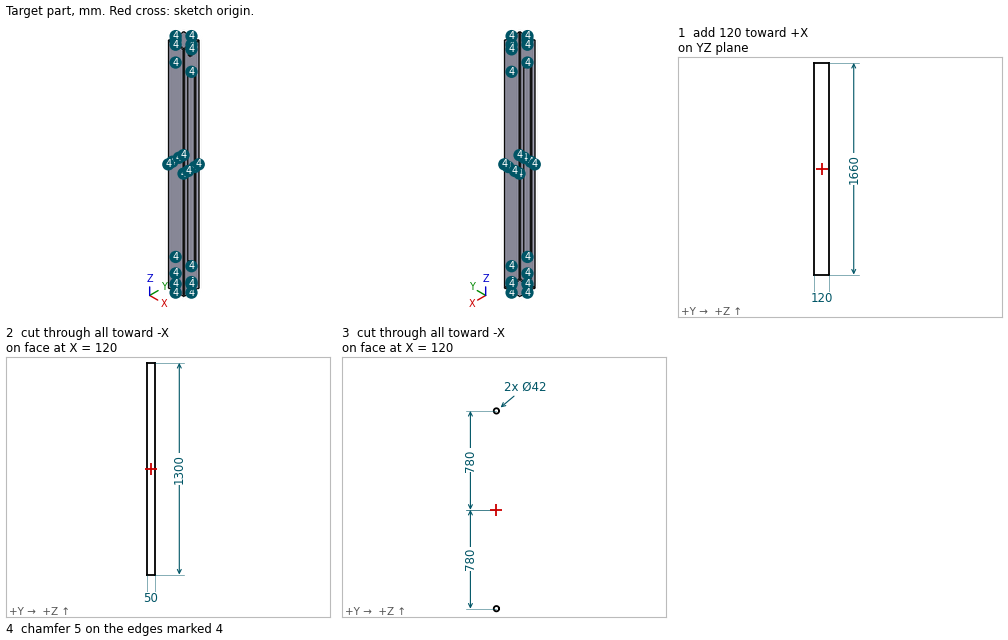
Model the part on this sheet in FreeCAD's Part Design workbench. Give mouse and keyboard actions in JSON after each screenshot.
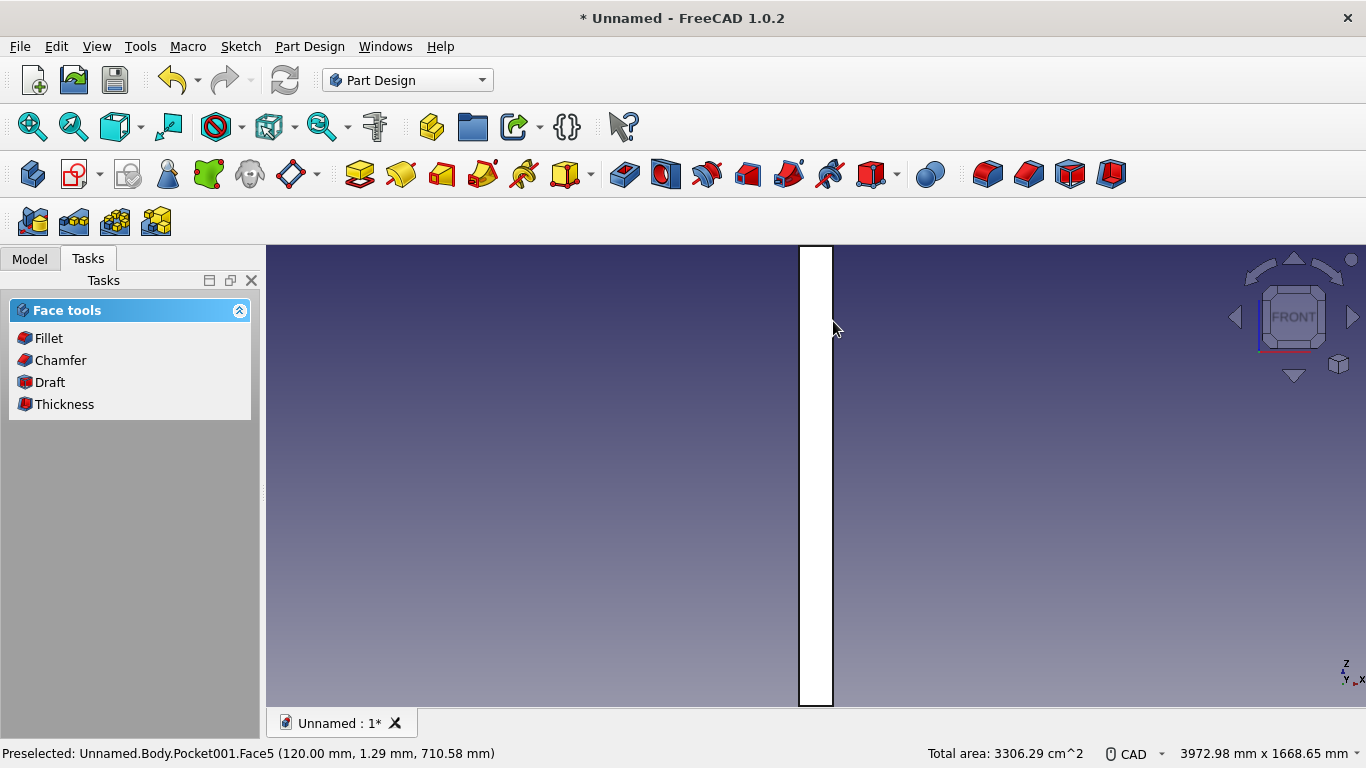
{"action": "key", "text": "3"}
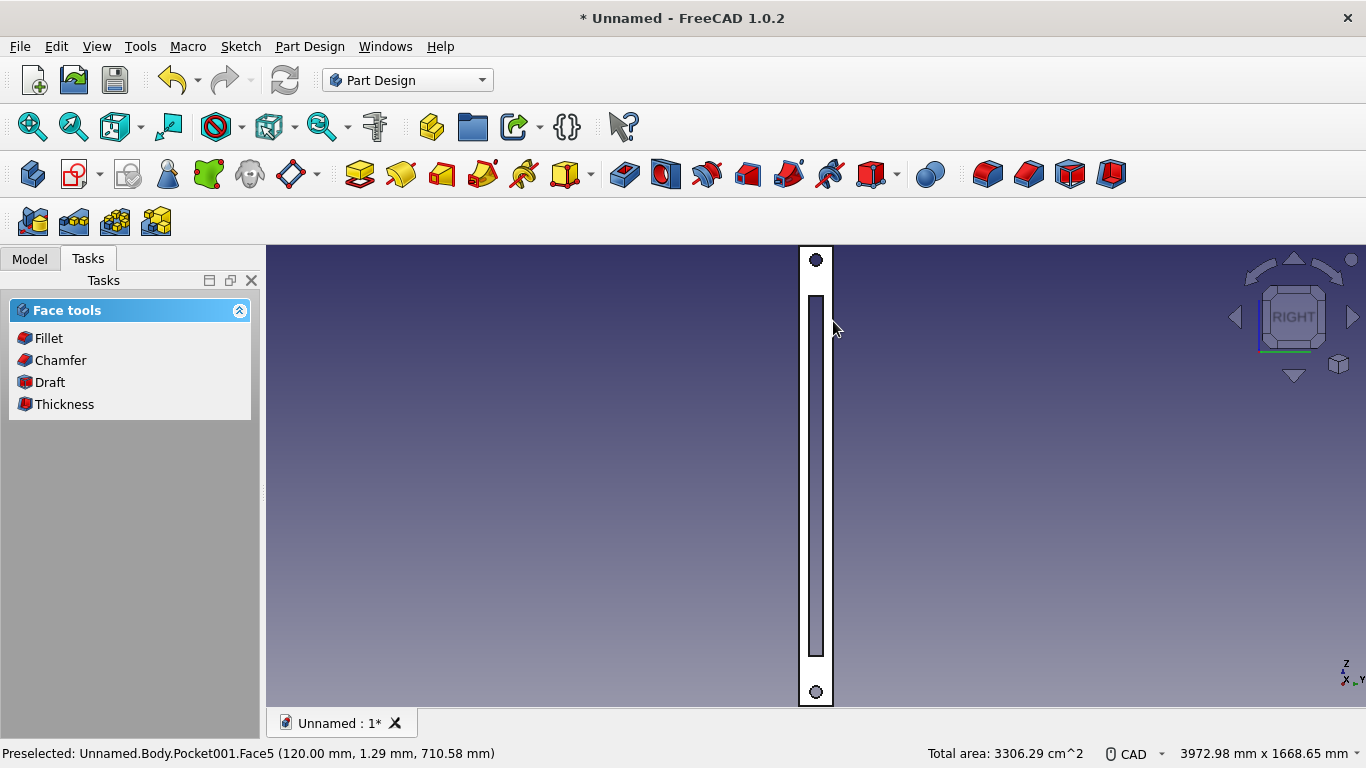
{"action": "key", "text": "5"}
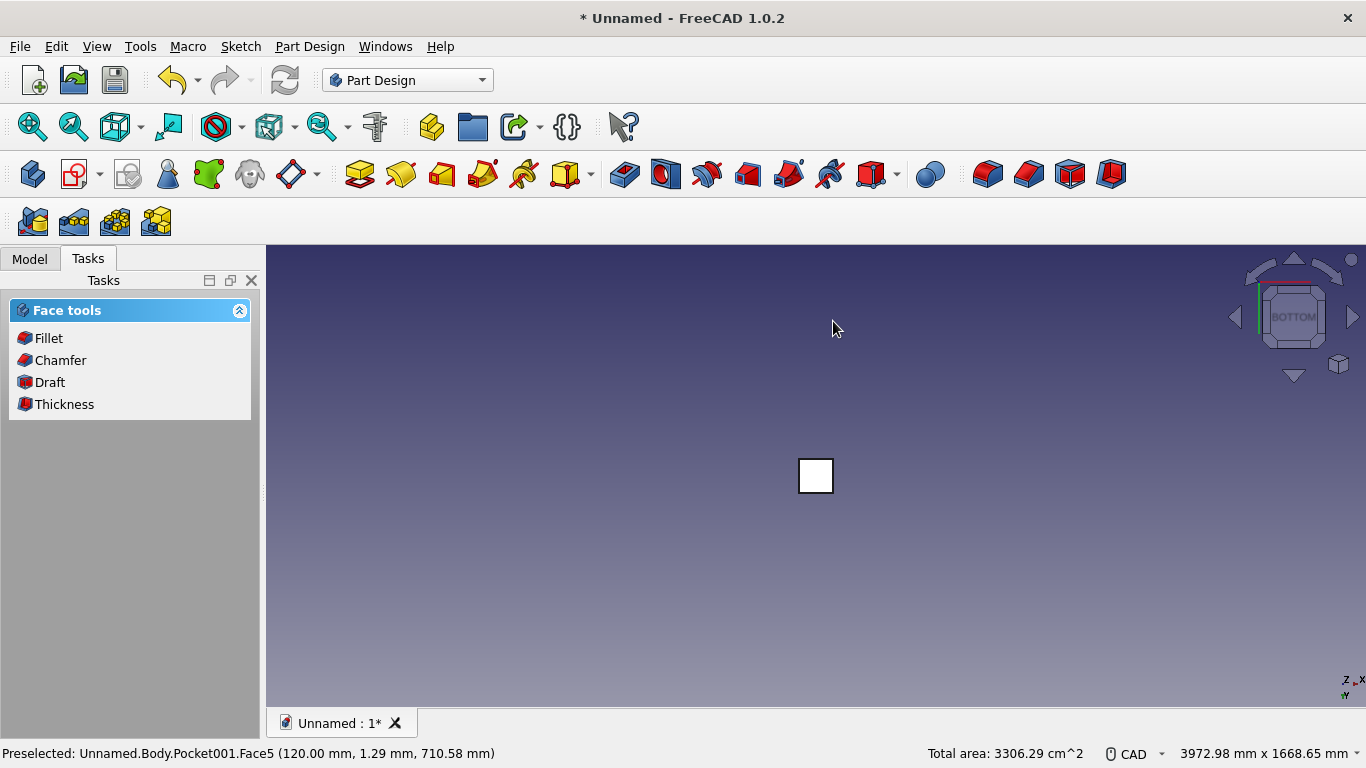
{"action": "left_click", "coordinate": [33, 128]}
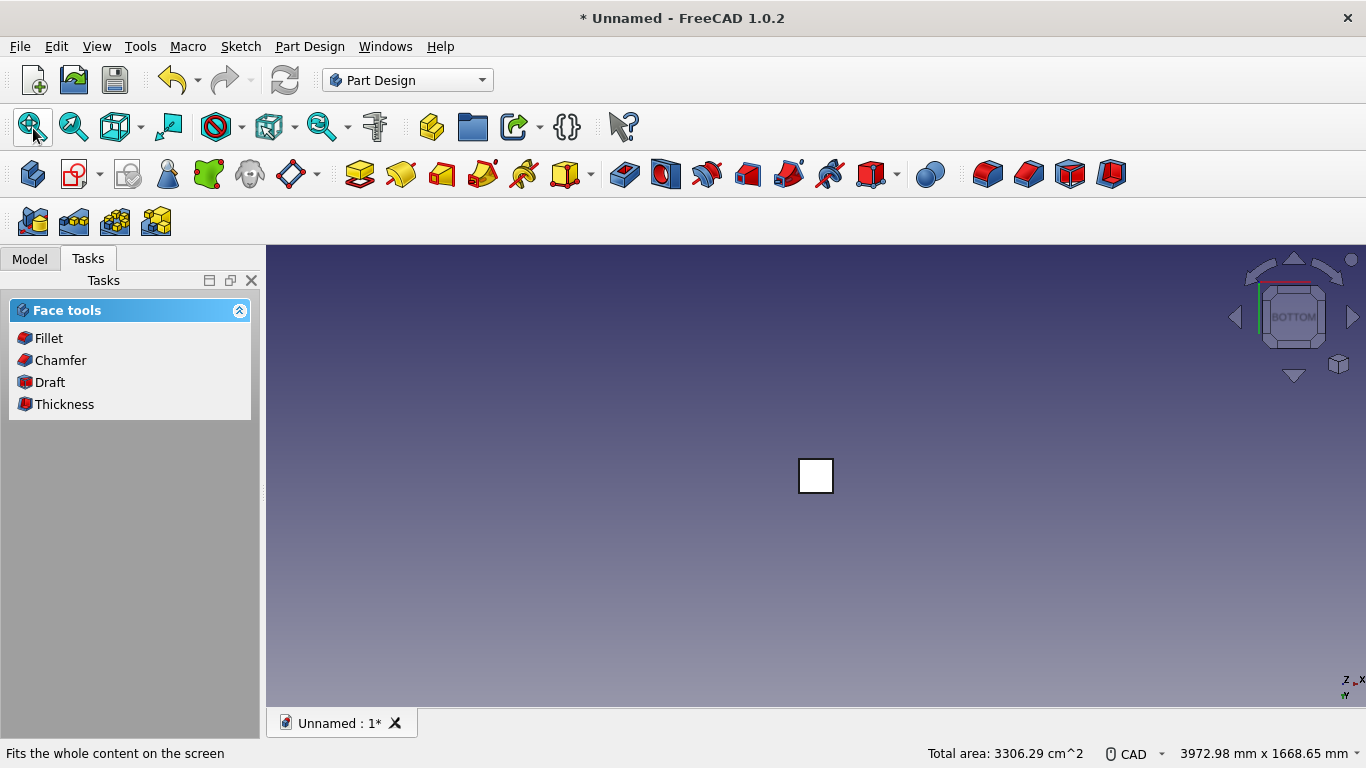
{"action": "key", "text": "4"}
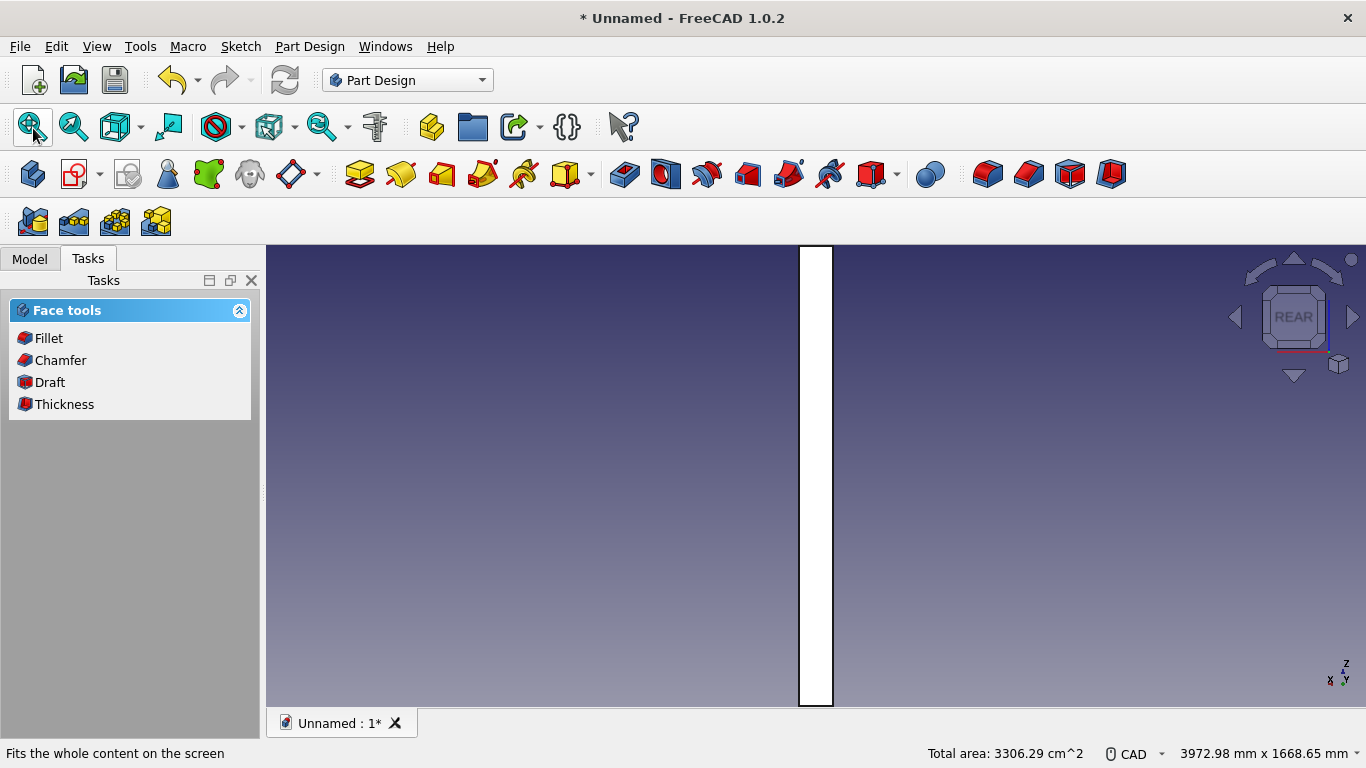
{"action": "left_click", "coordinate": [816, 672], "text": "ctrl"}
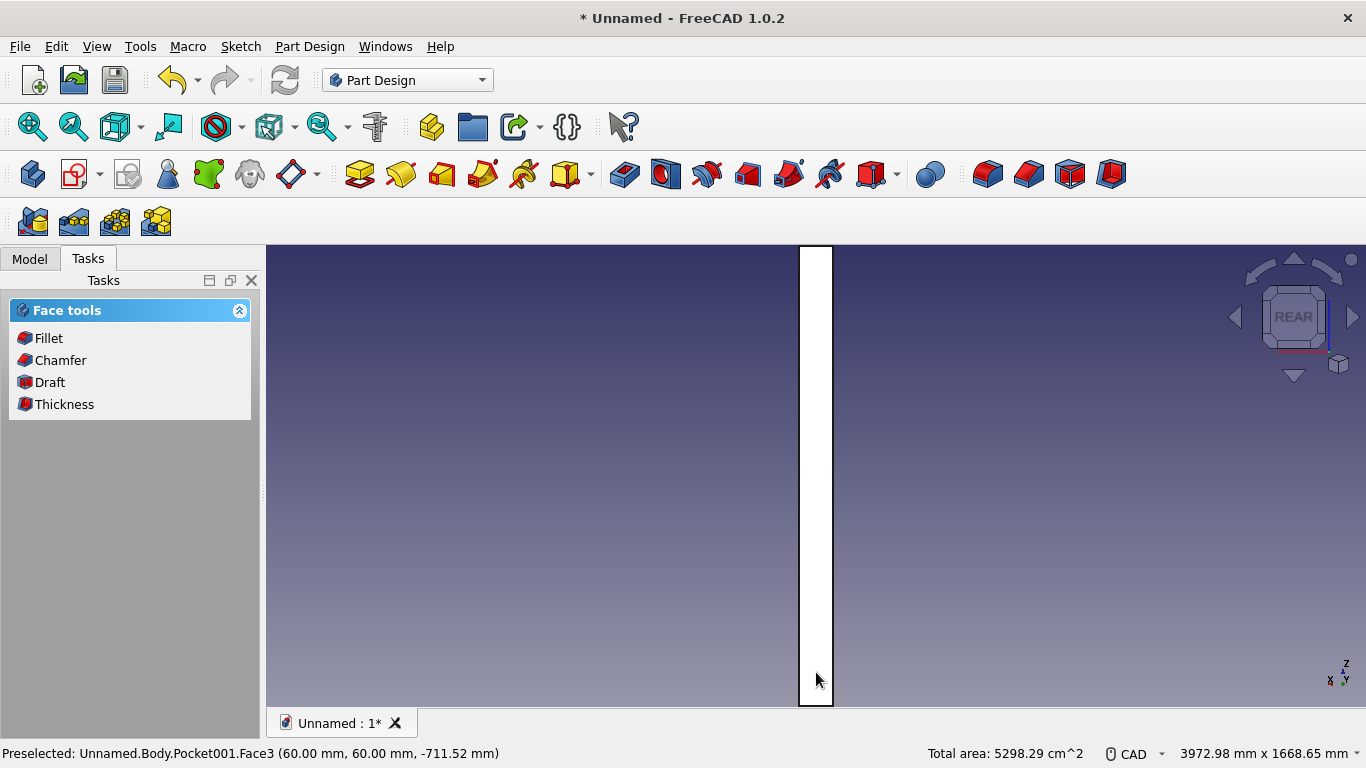
{"action": "key", "text": "6"}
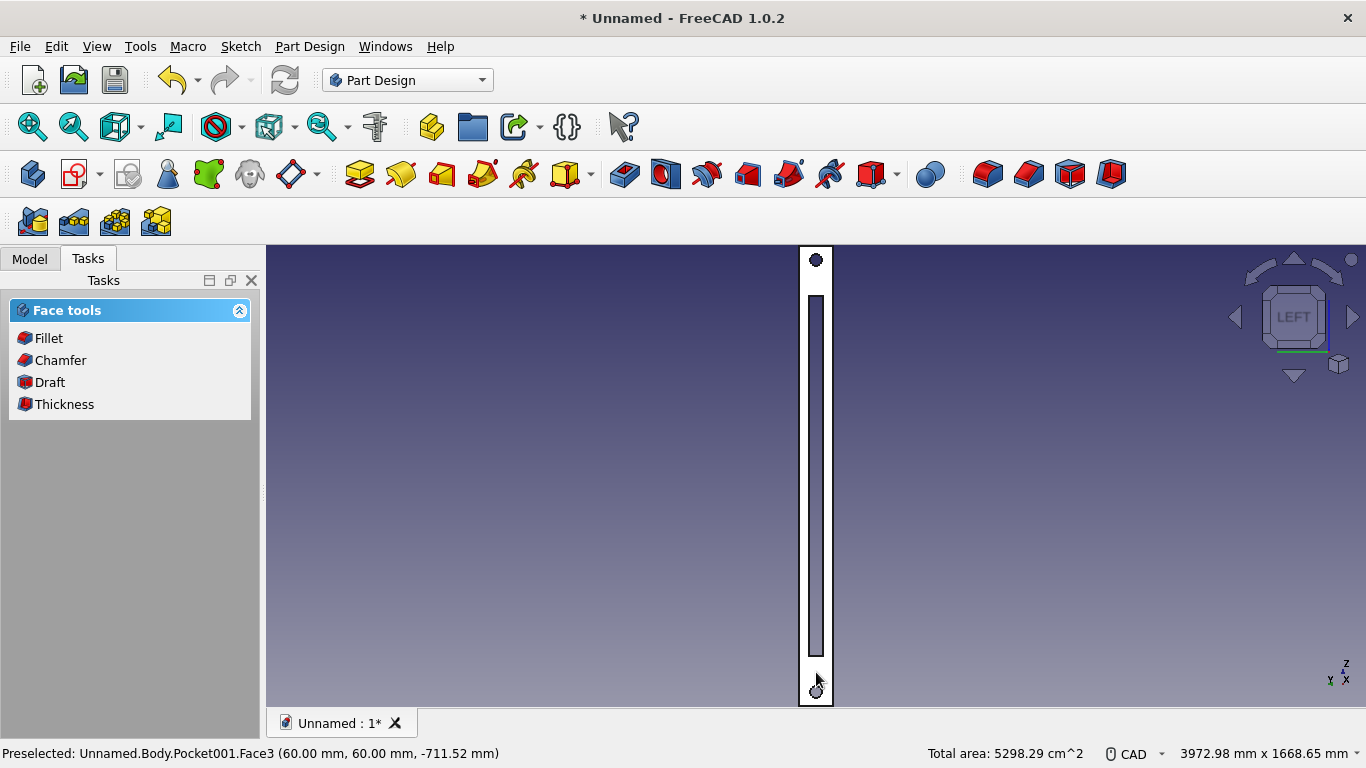
{"action": "left_click", "coordinate": [816, 278], "text": "ctrl"}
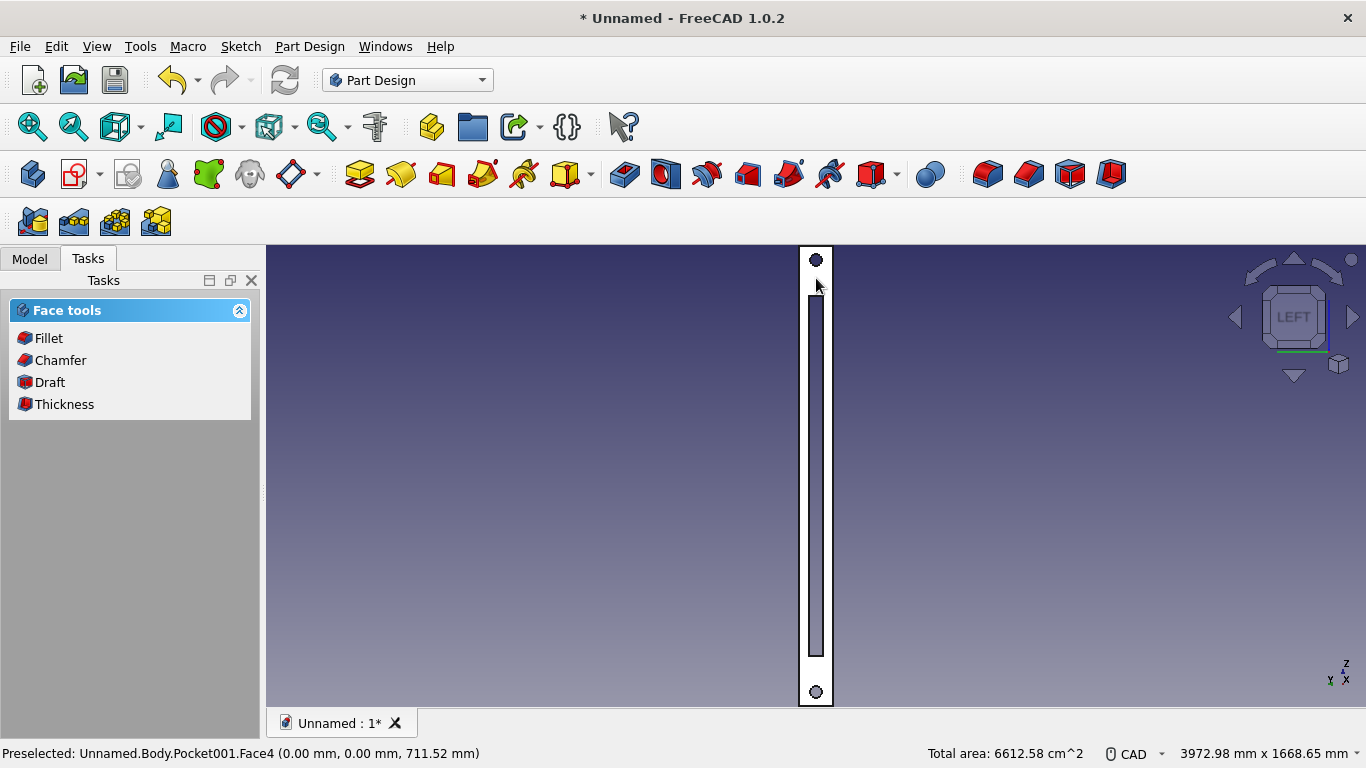
{"action": "left_click", "coordinate": [1029, 174]}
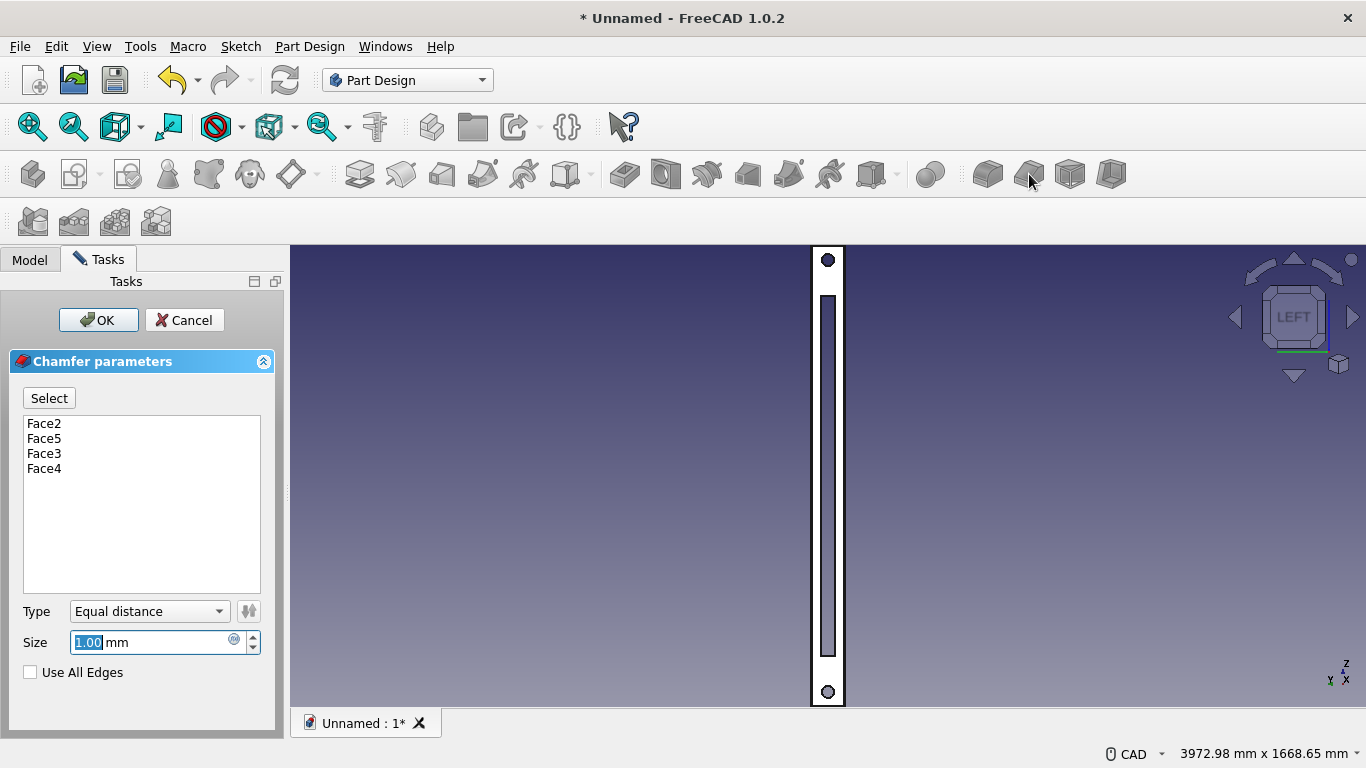
{"action": "type", "text": "5"}
{"action": "key", "text": "Tab"}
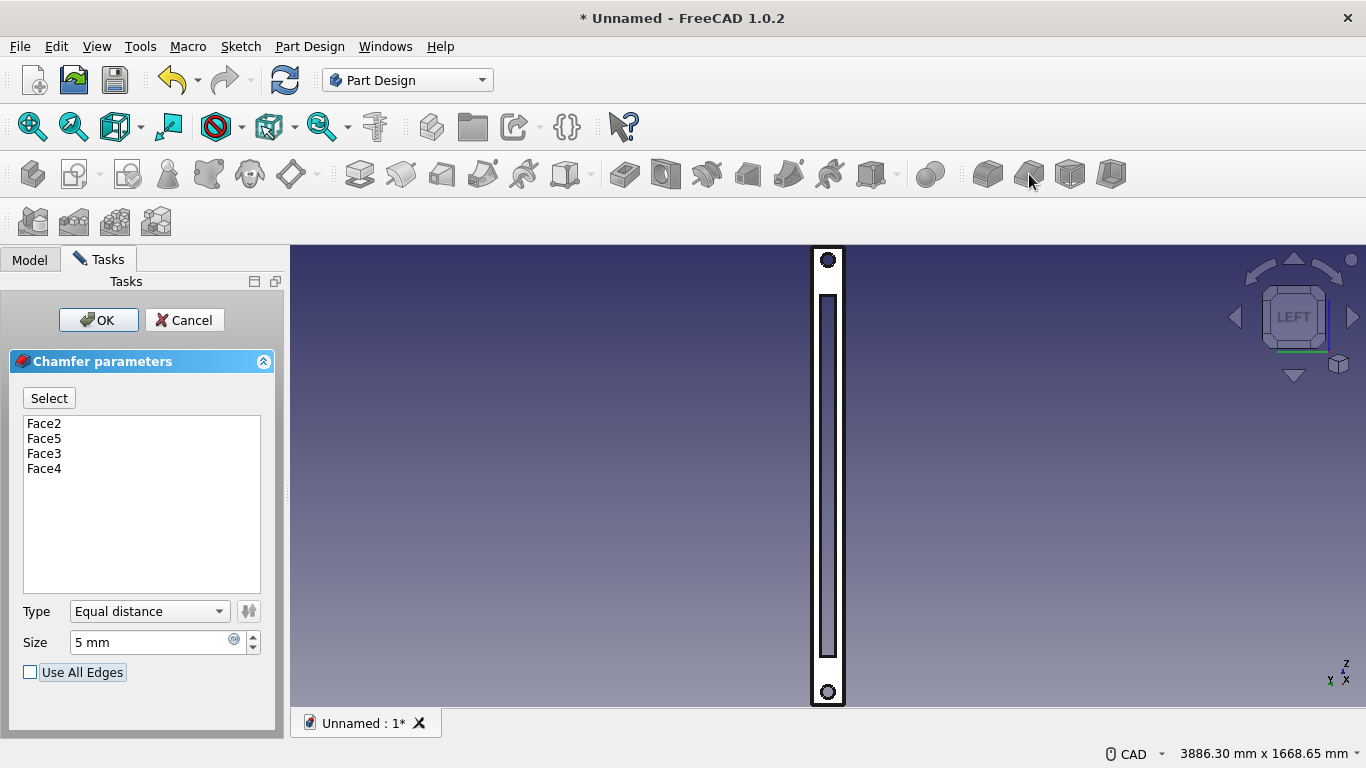
{"action": "left_click", "coordinate": [99, 320]}